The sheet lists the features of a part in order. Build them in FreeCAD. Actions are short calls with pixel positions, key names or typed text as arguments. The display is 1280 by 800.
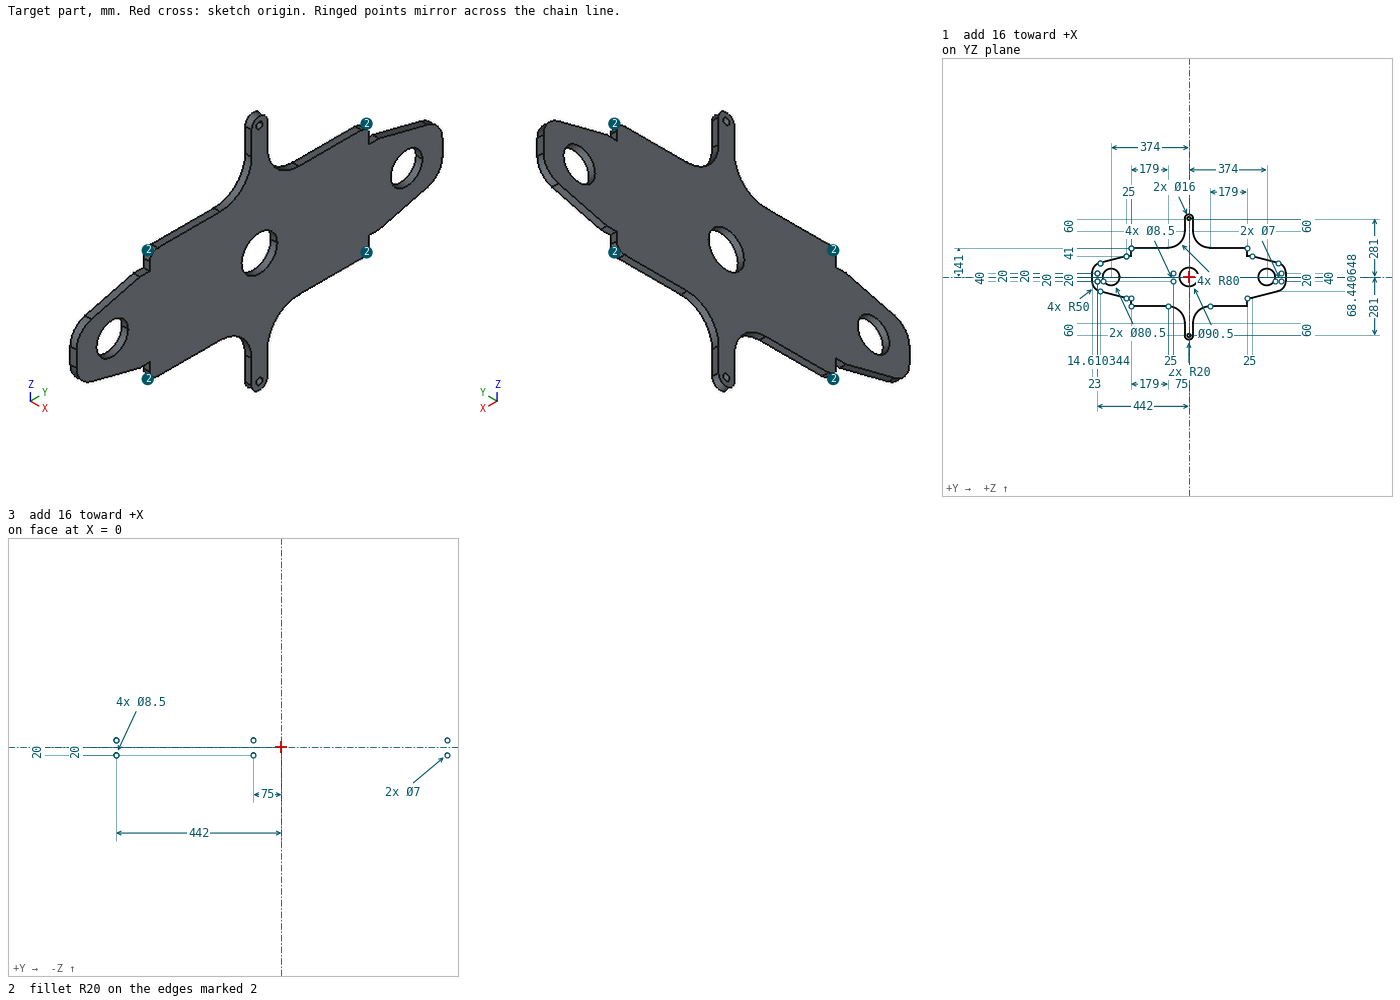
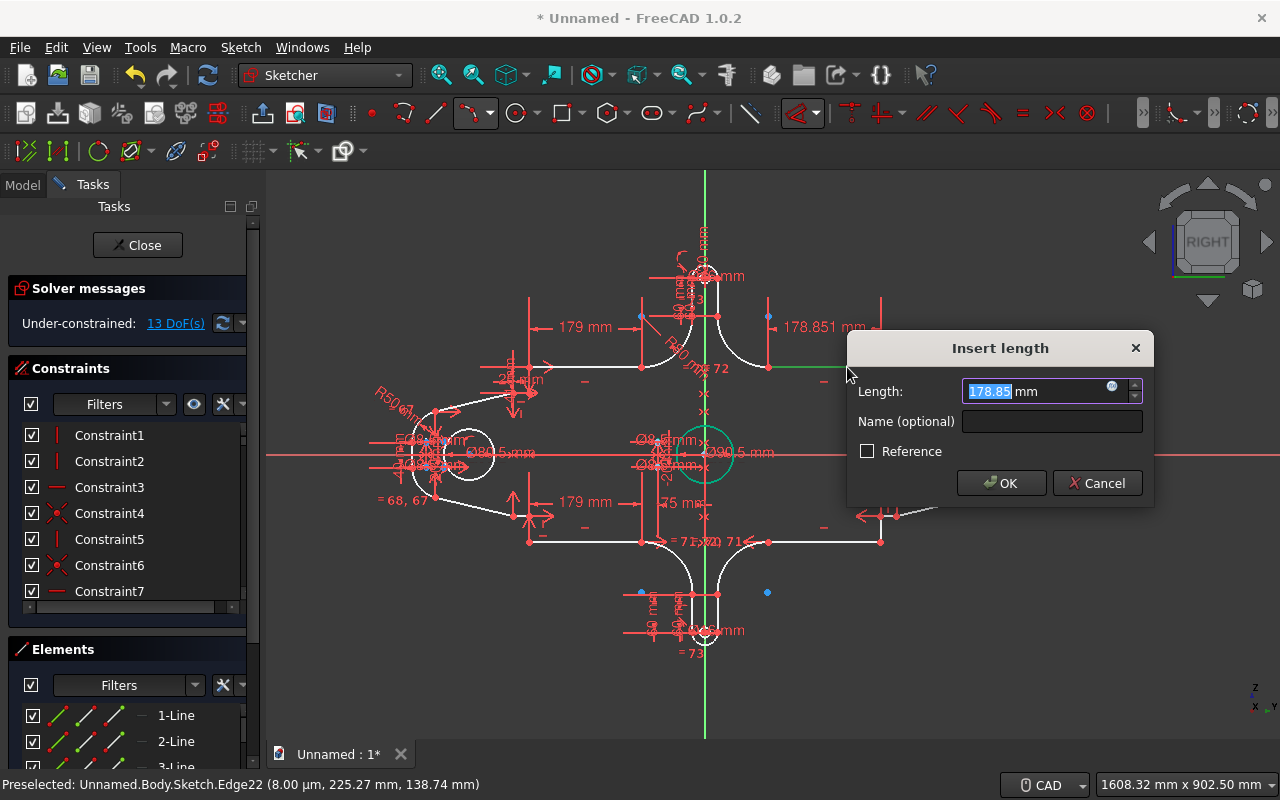
text(179)
key(Return)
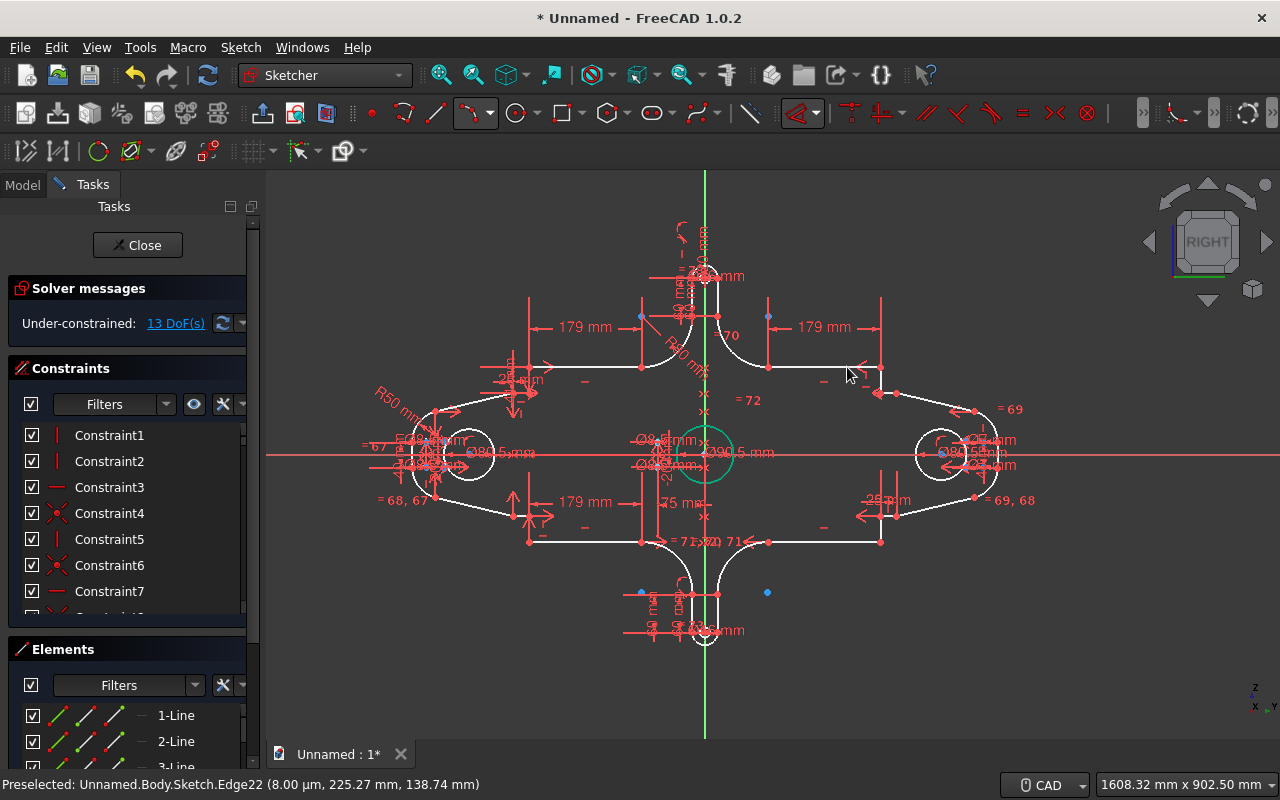
scroll(412, 443, up, 6)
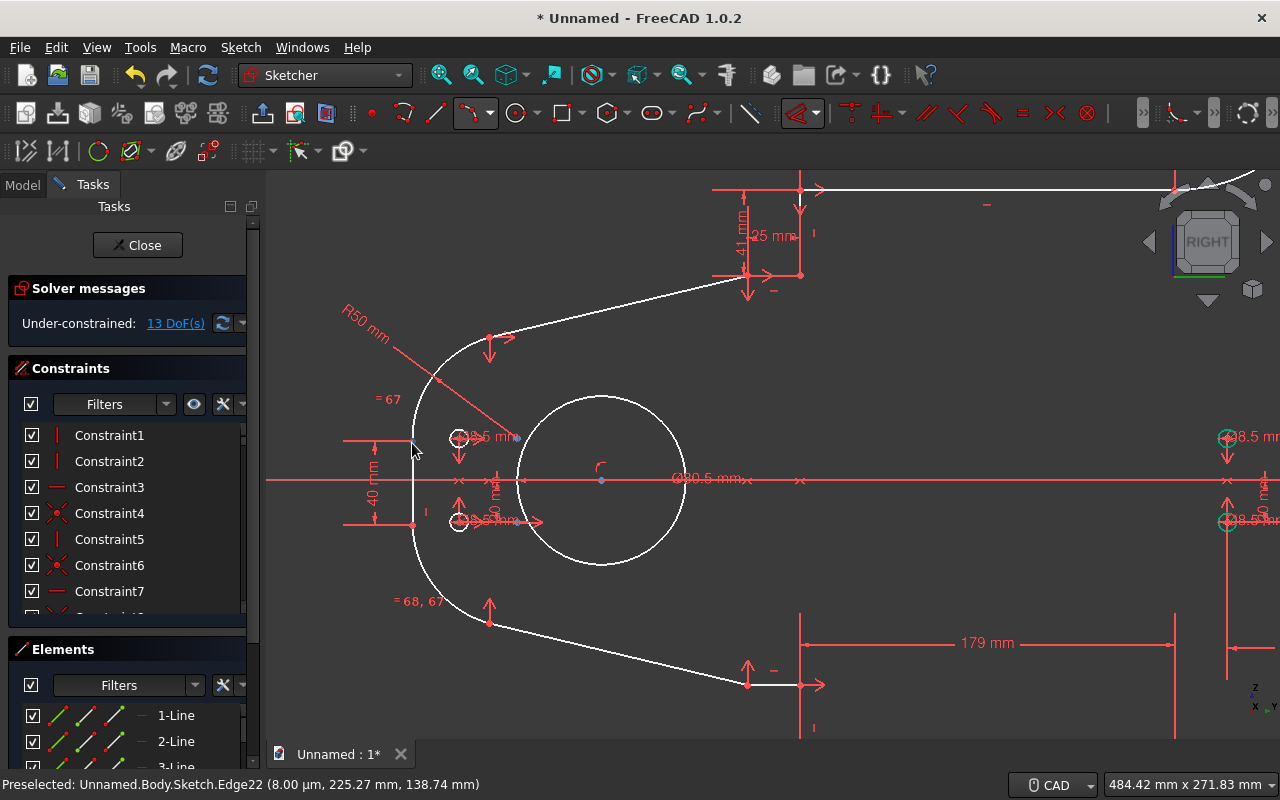
click(413, 441)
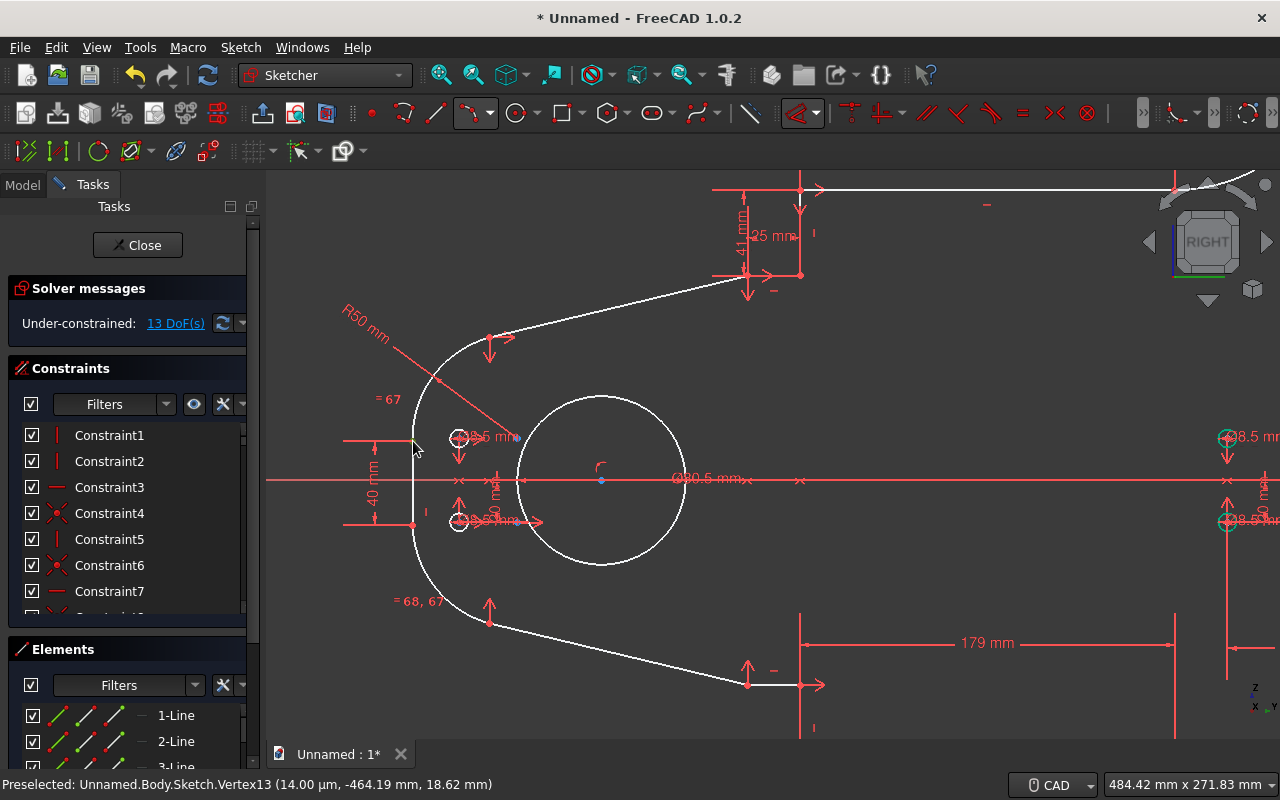
click(818, 114)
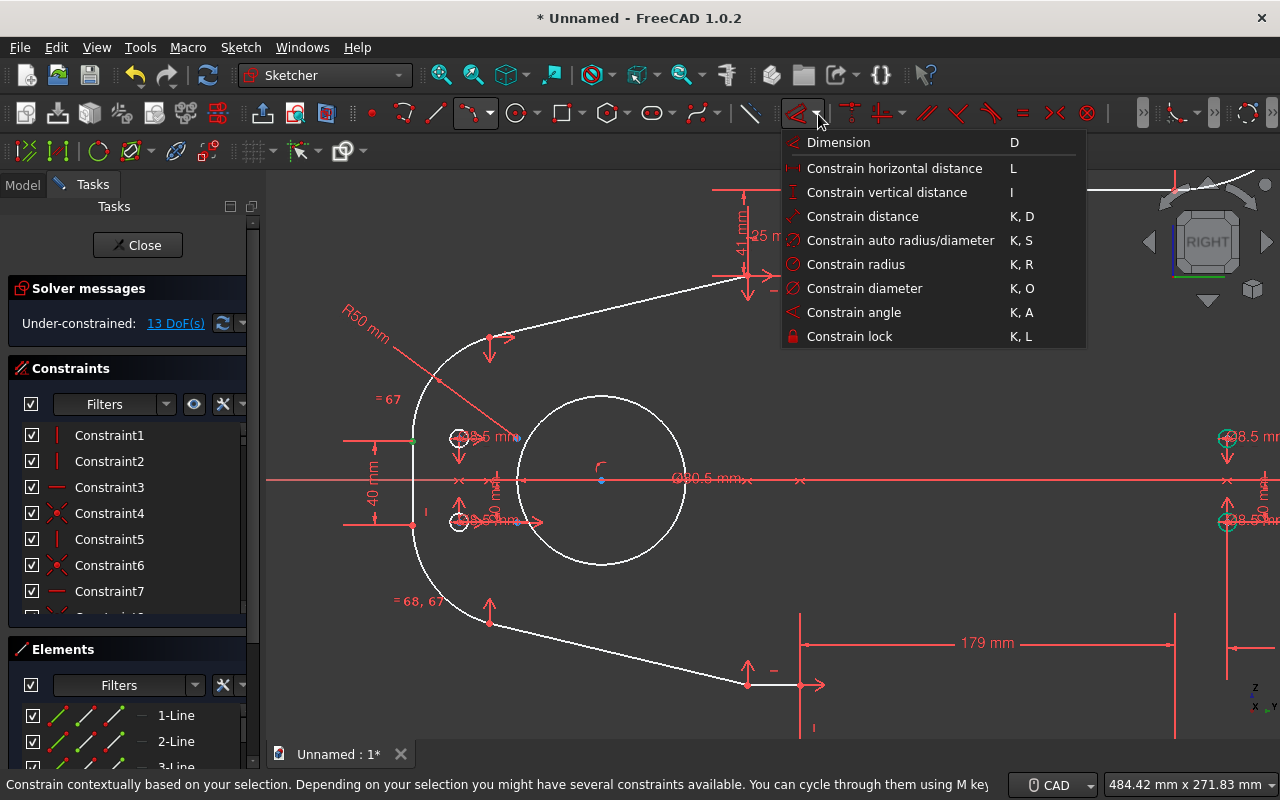
click(934, 192)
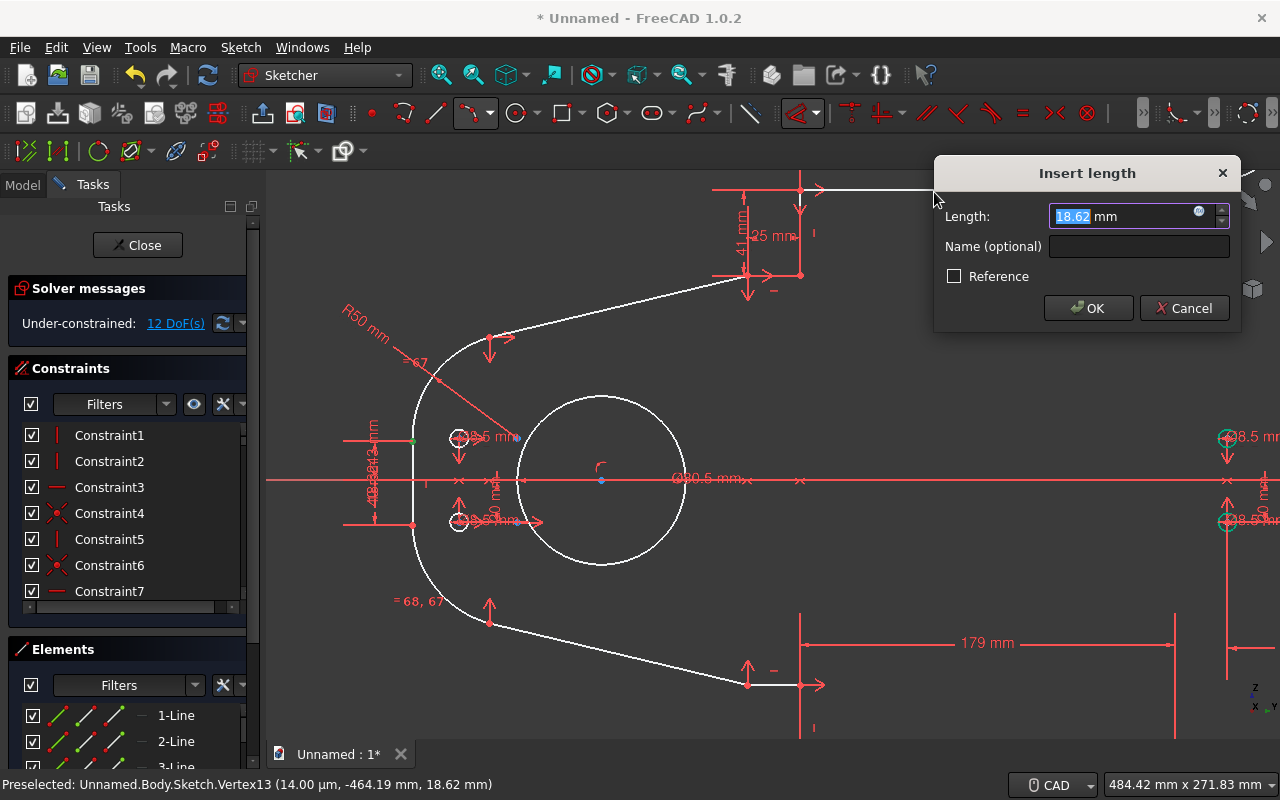
text(20)
key(Return)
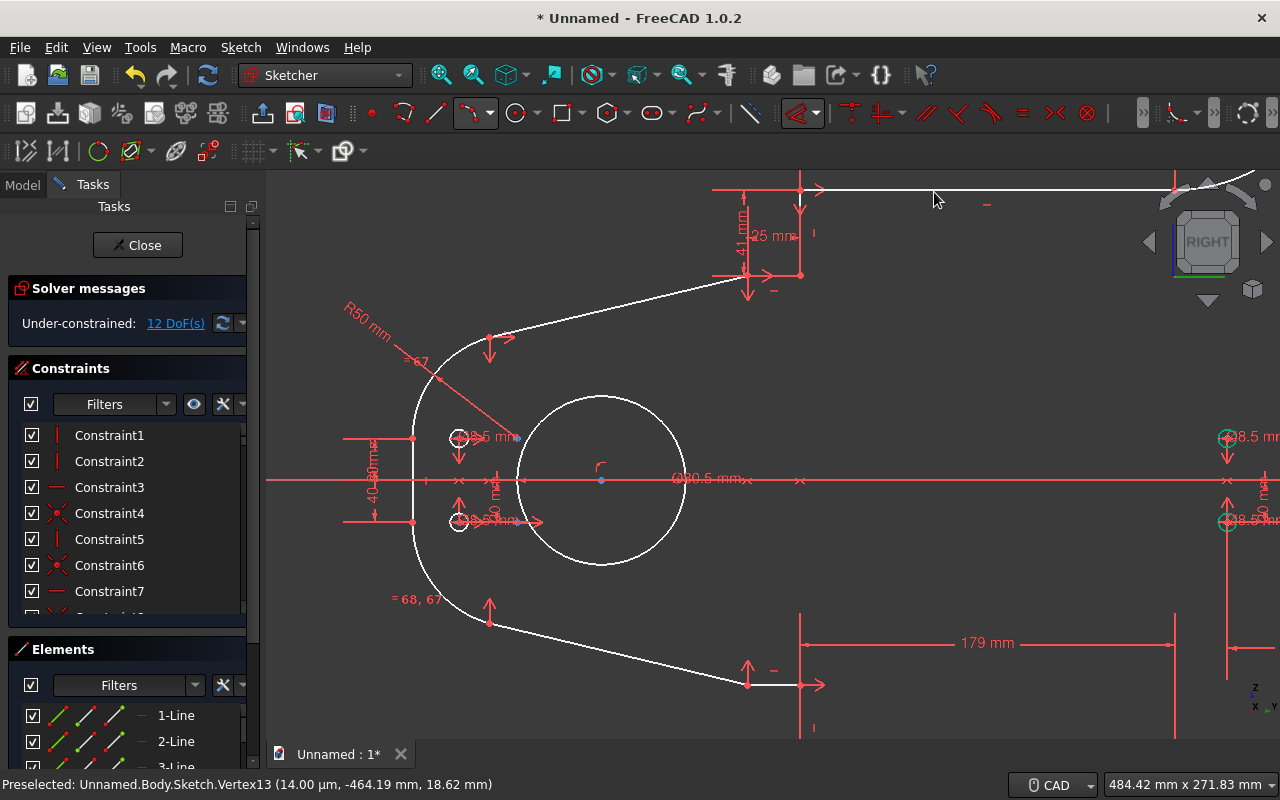
scroll(411, 443, down, 6)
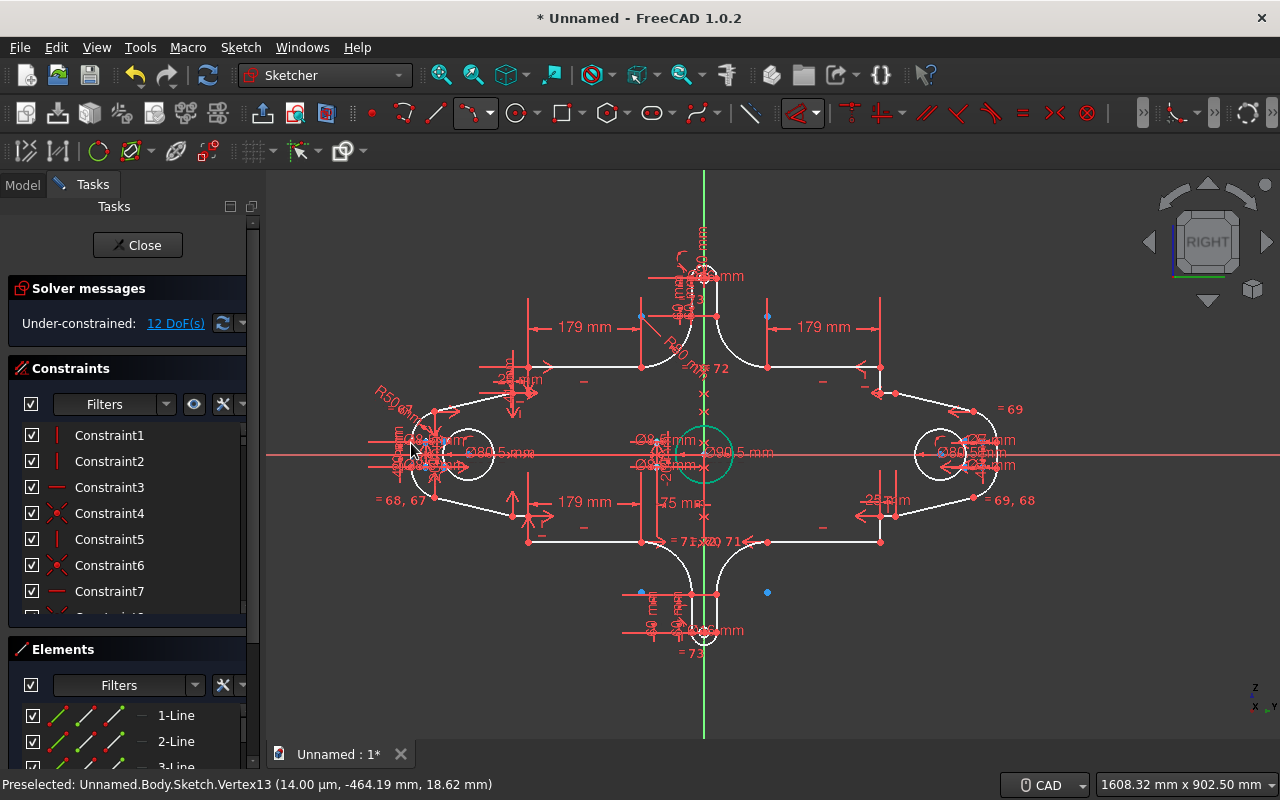
scroll(997, 468, up, 6)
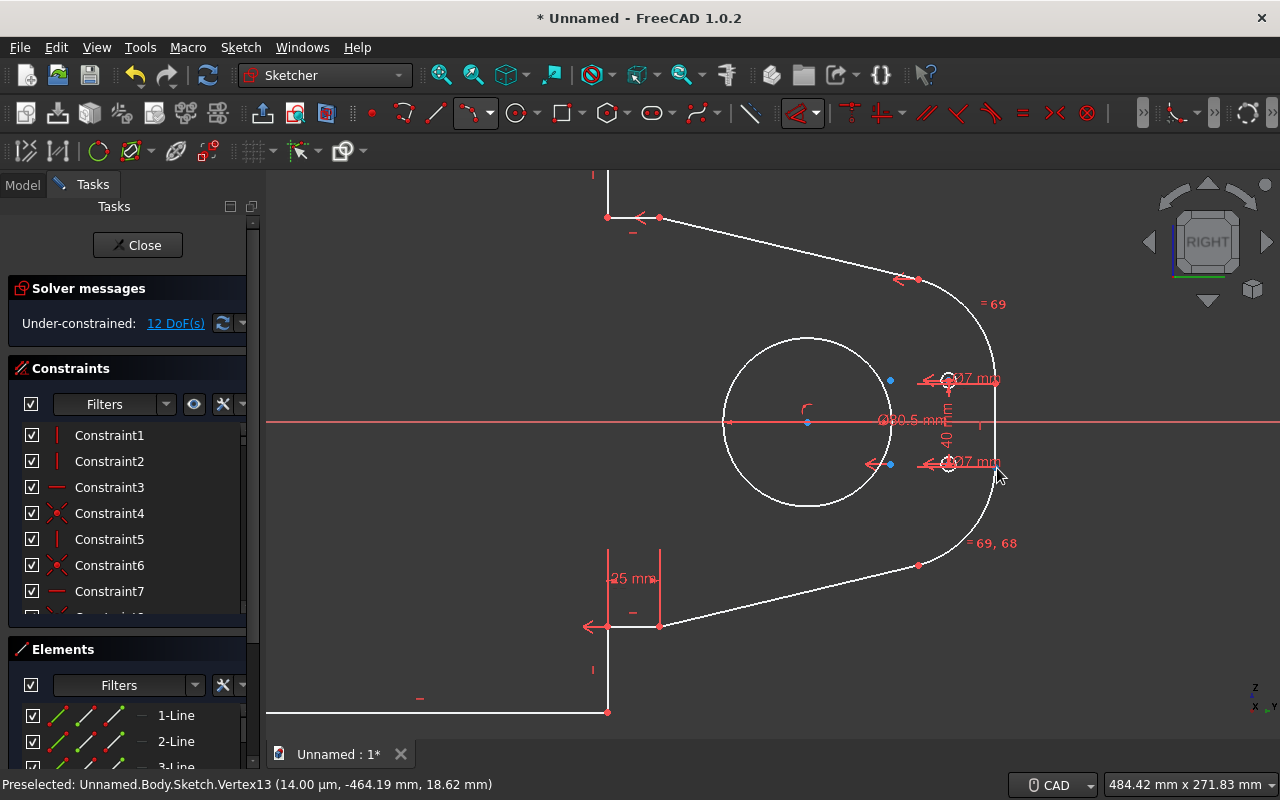
click(995, 467)